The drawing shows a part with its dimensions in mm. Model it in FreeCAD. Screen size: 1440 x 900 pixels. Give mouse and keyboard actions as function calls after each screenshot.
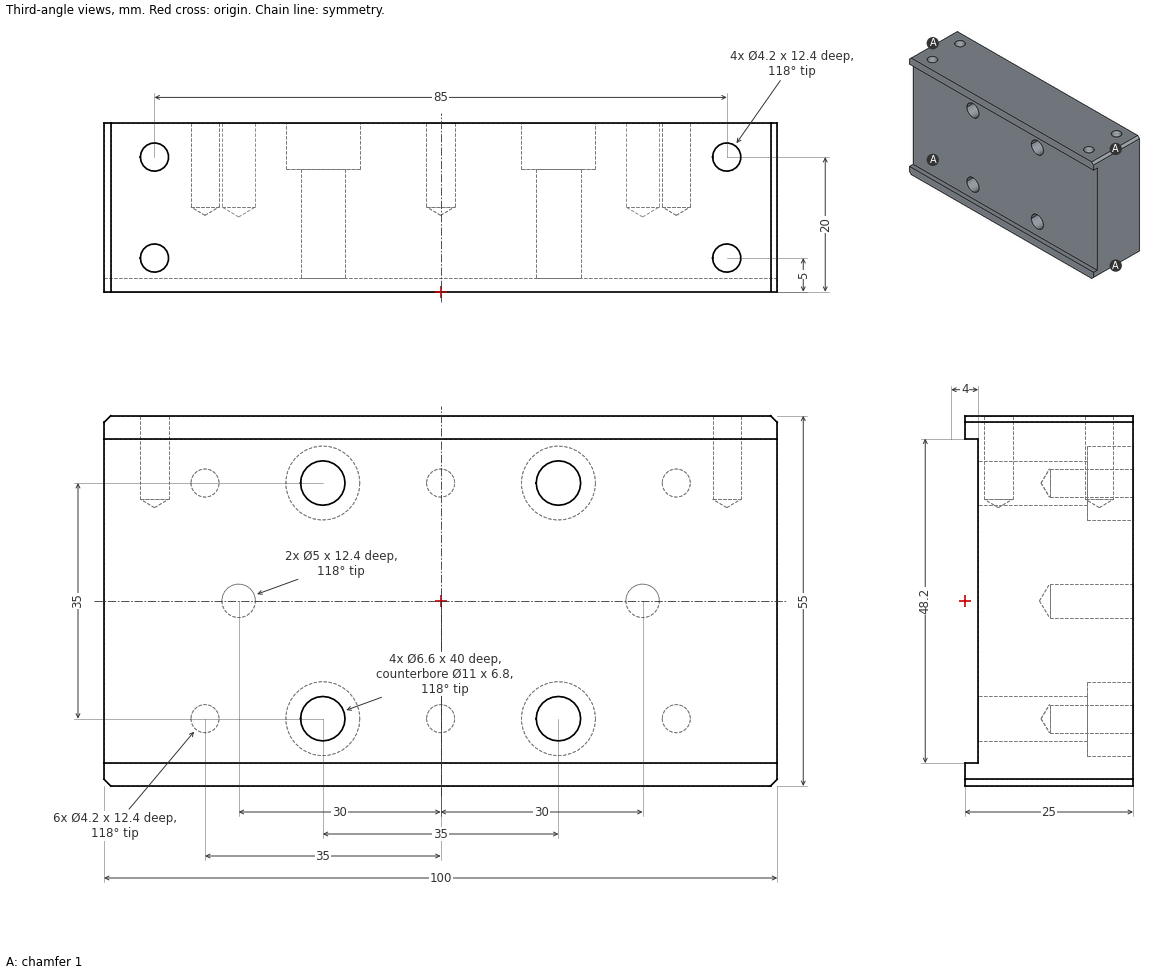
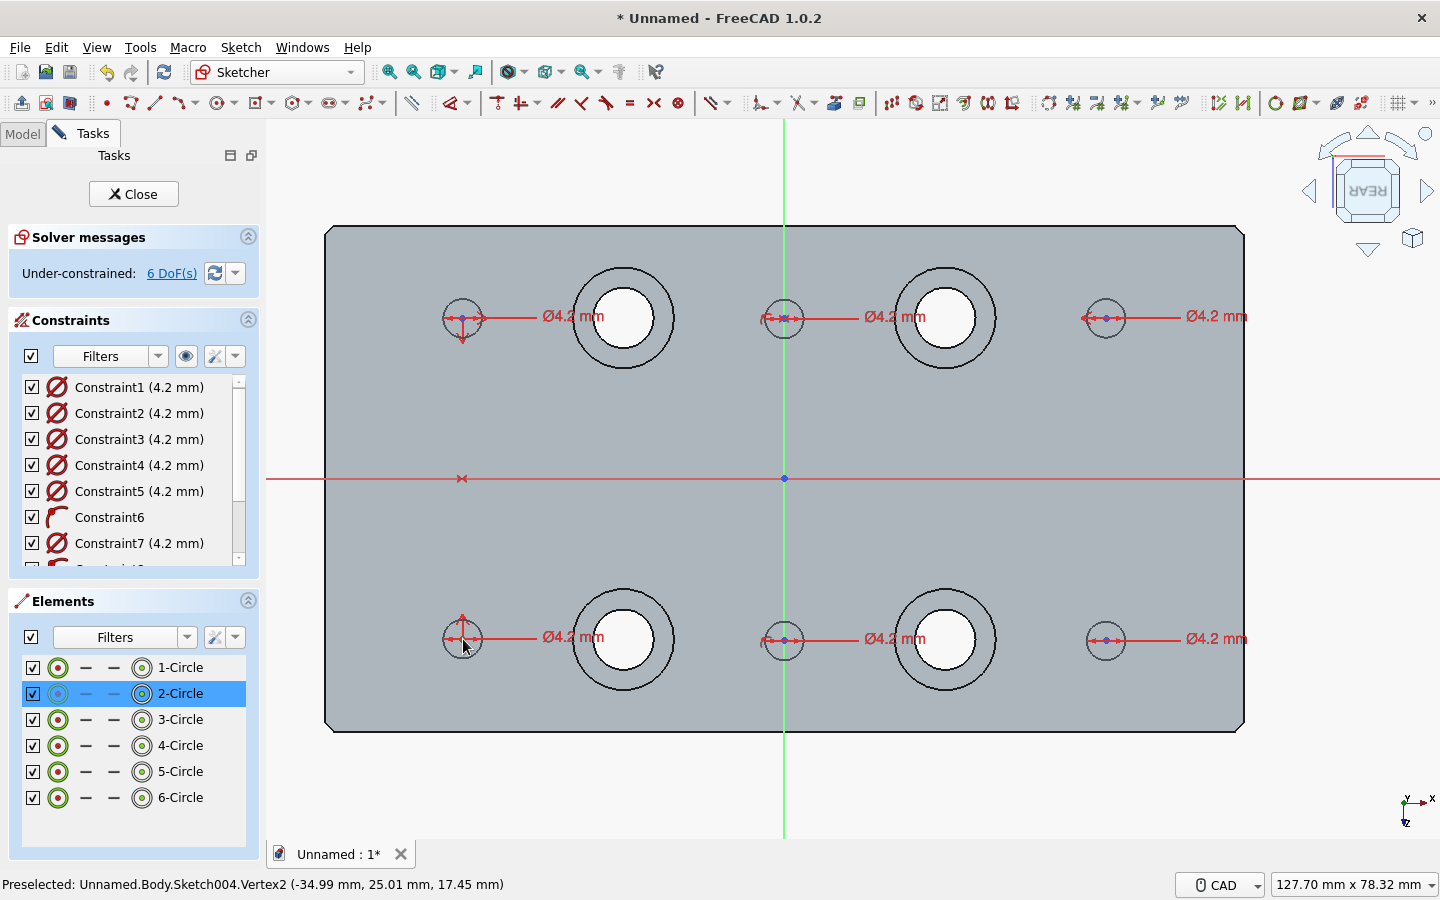
click(1106, 641)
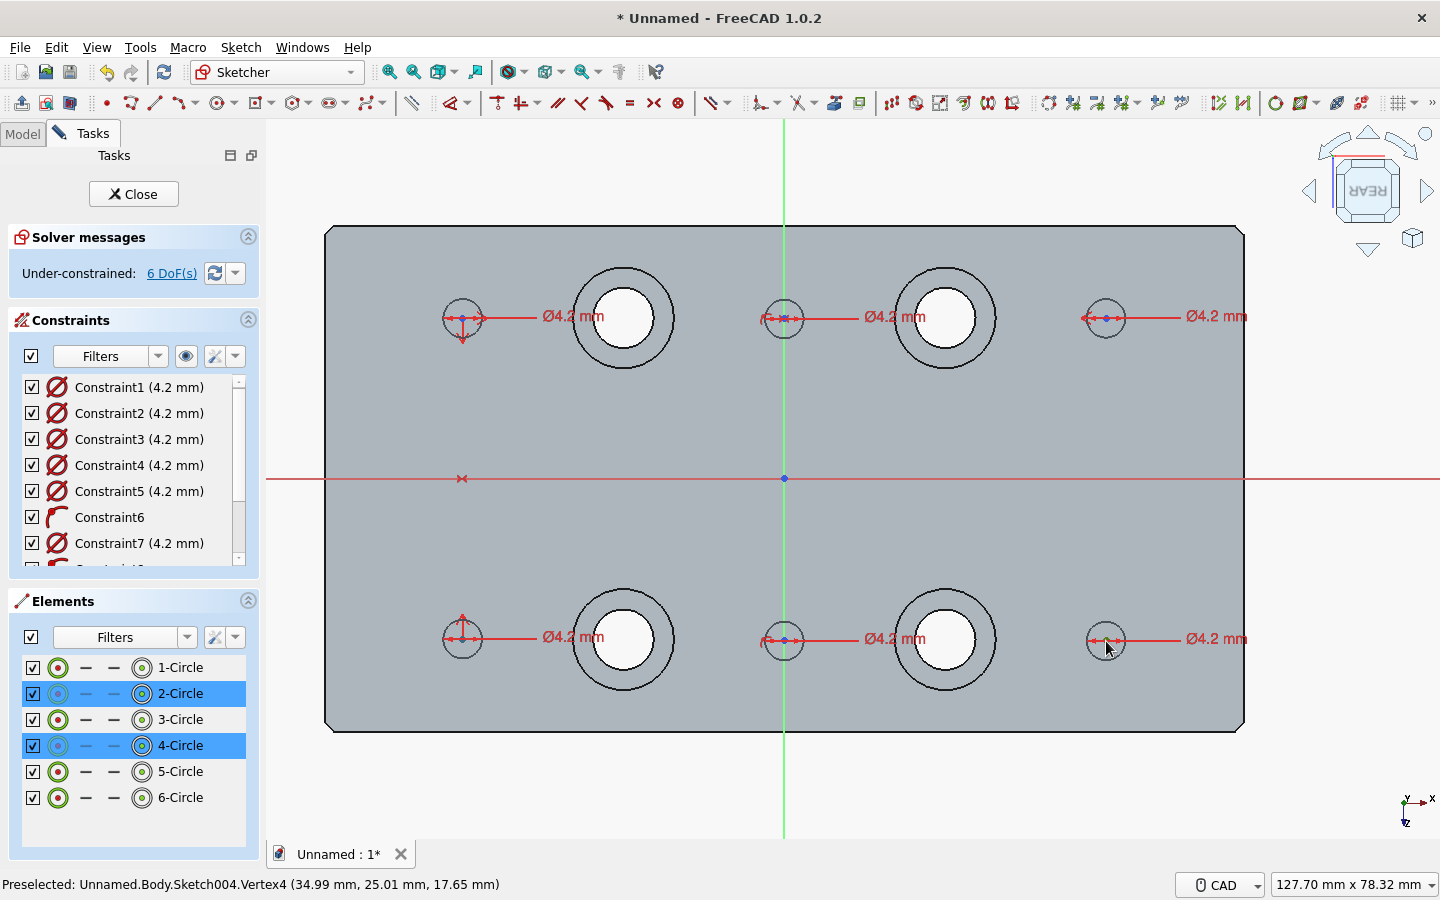
click(784, 764)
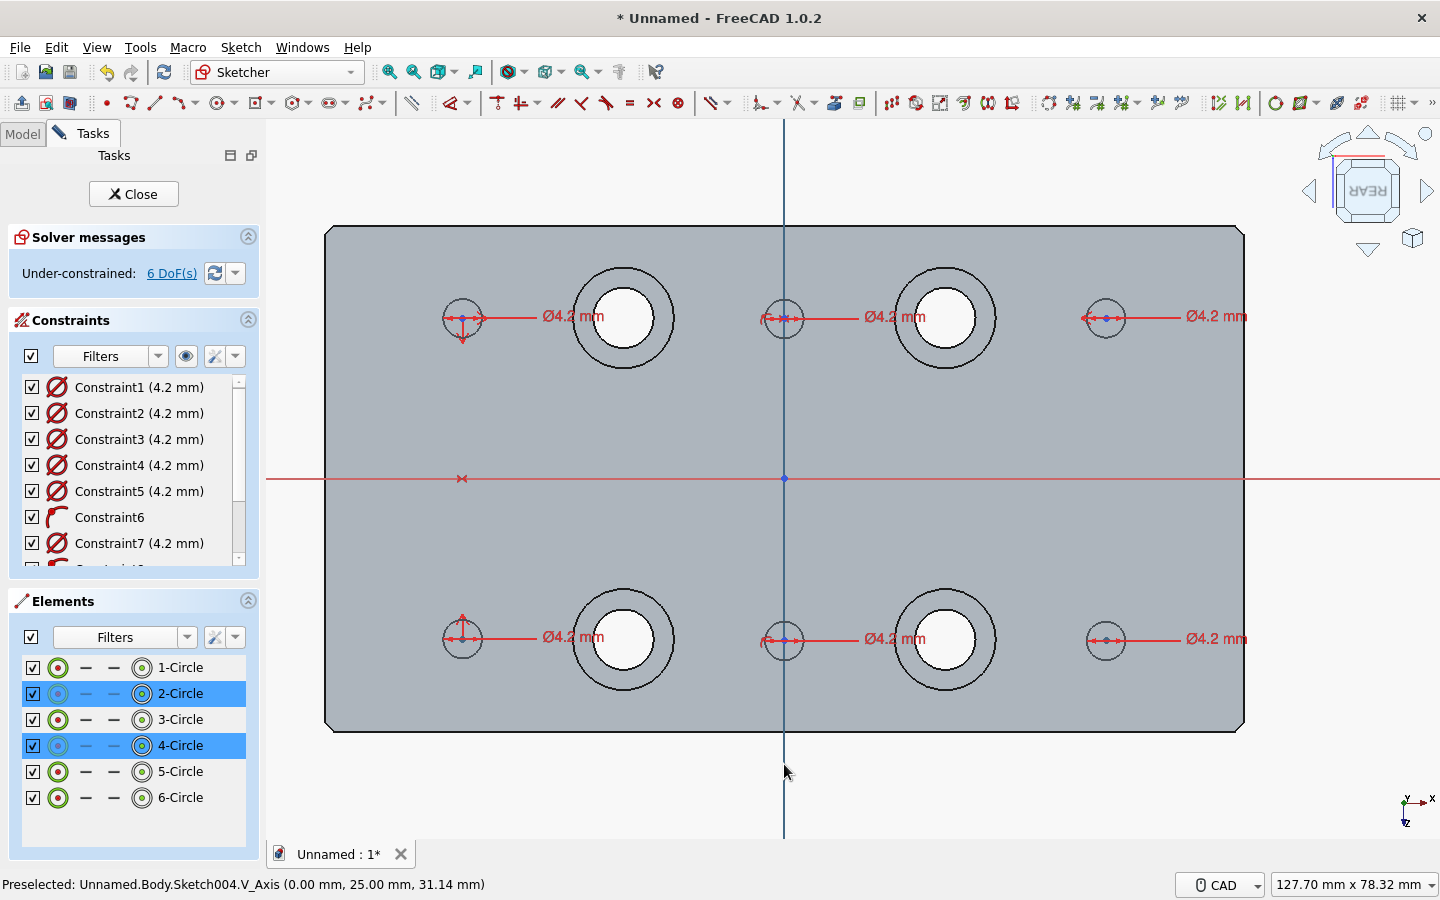
click(654, 104)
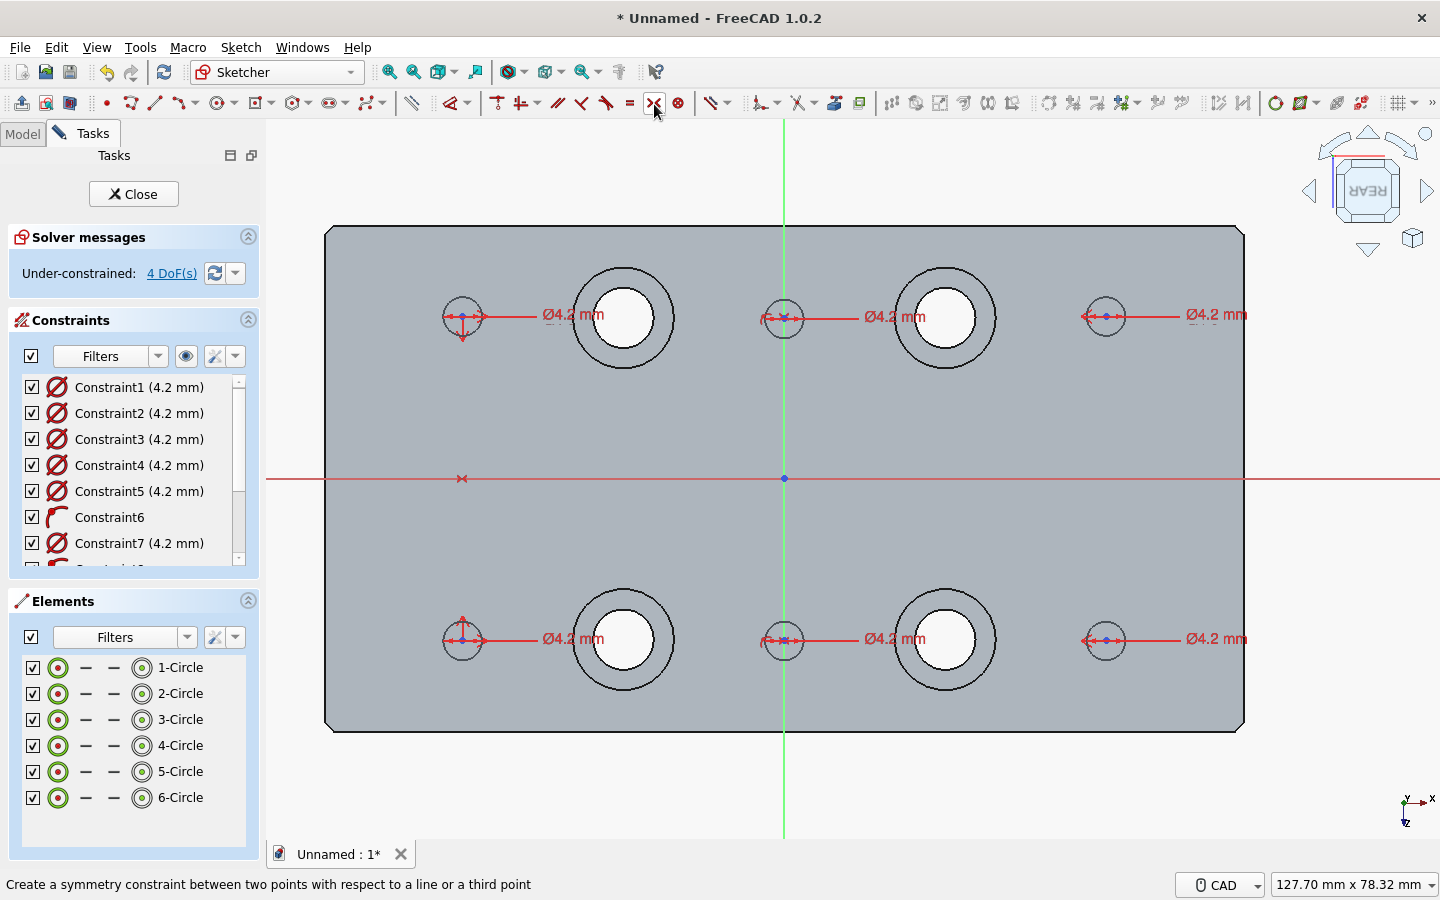
click(450, 104)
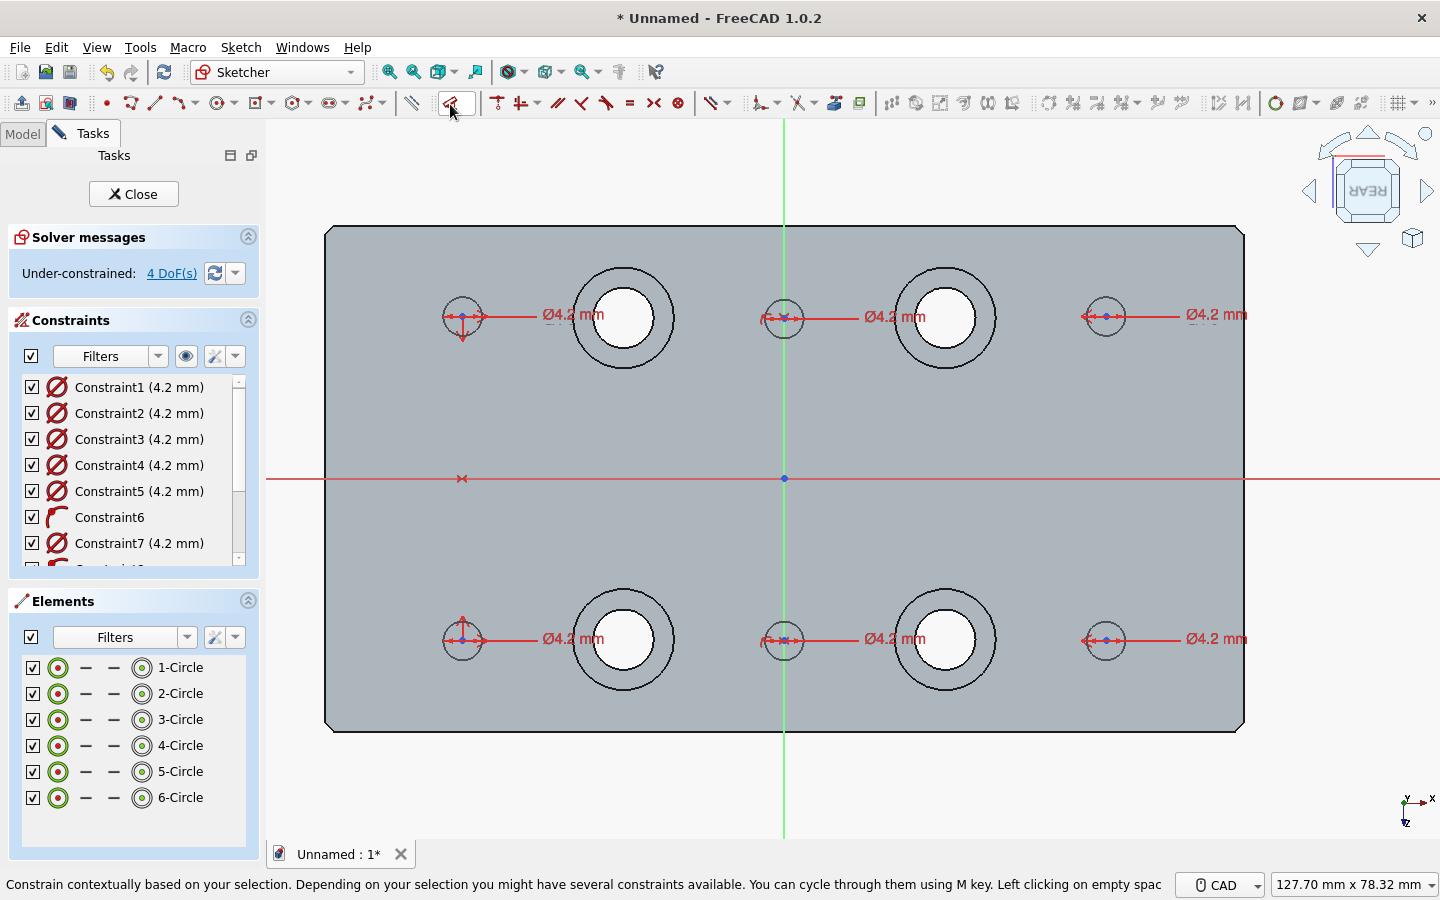
click(463, 317)
click(623, 283)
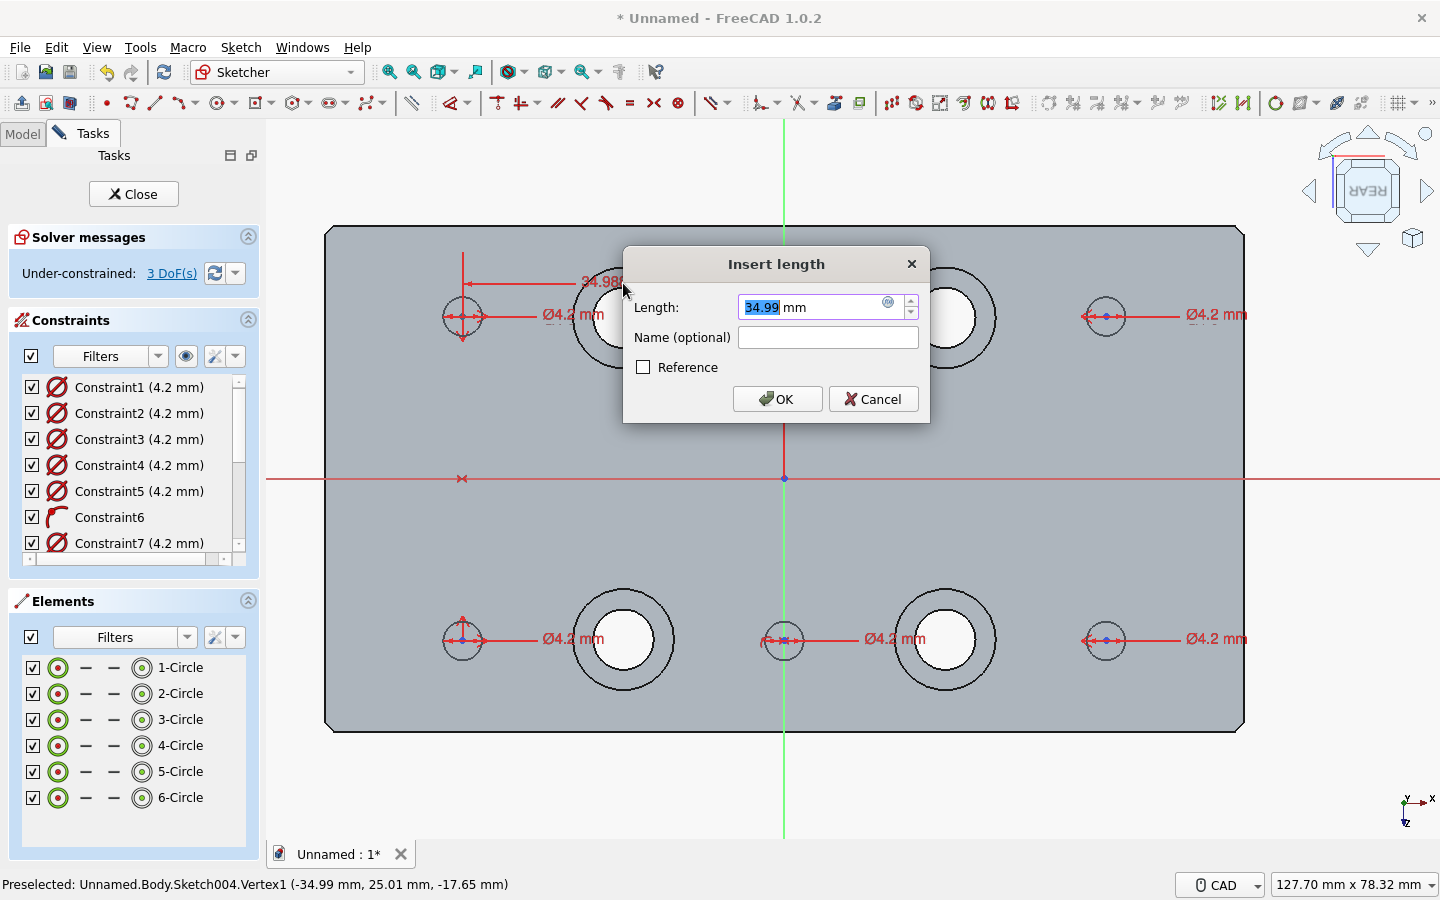
text(35)
key(Return)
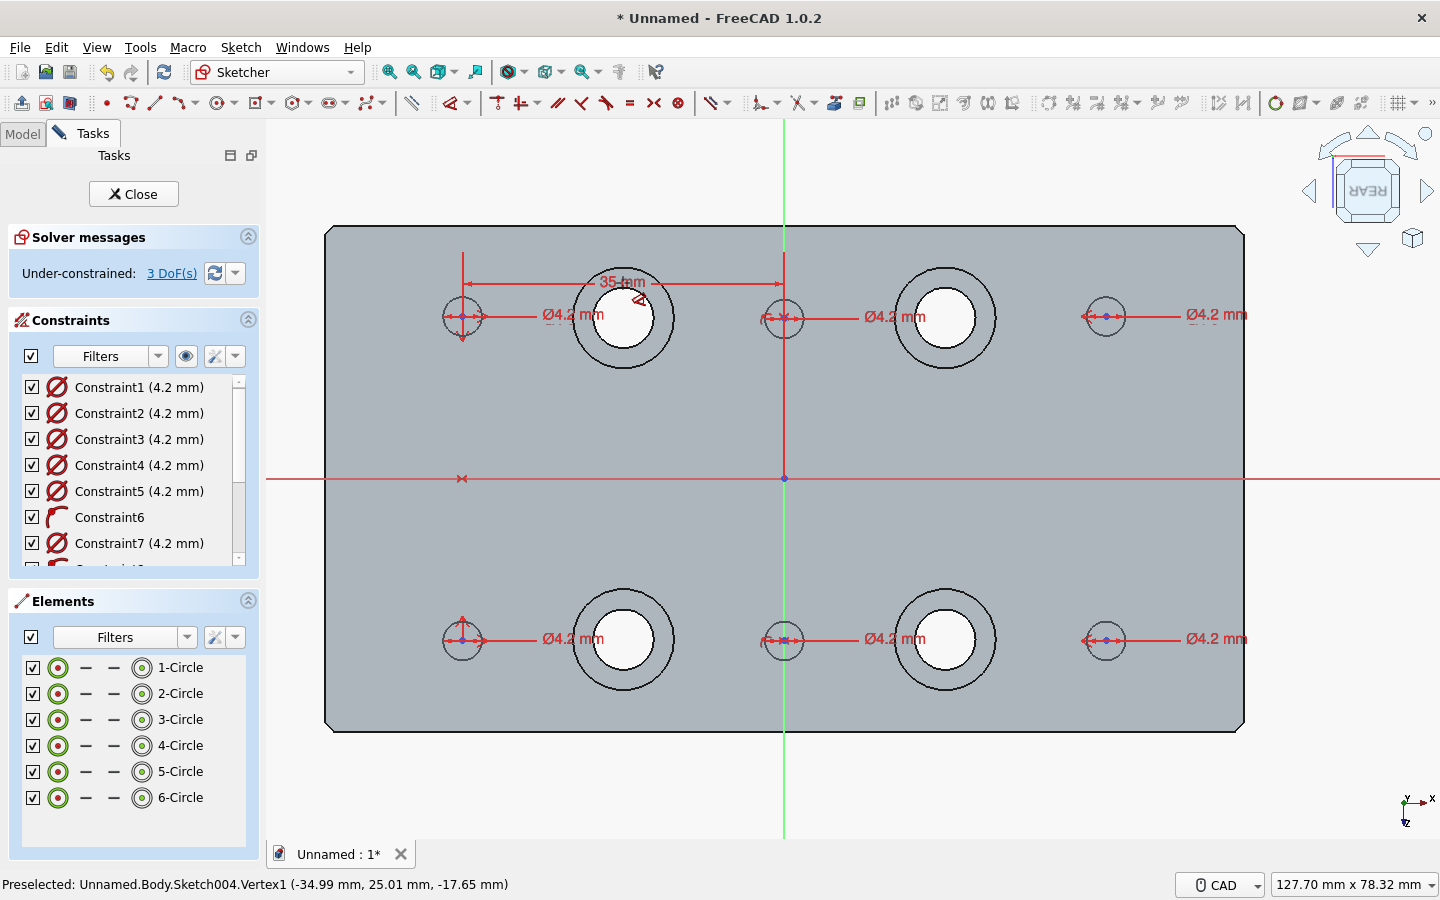
click(463, 317)